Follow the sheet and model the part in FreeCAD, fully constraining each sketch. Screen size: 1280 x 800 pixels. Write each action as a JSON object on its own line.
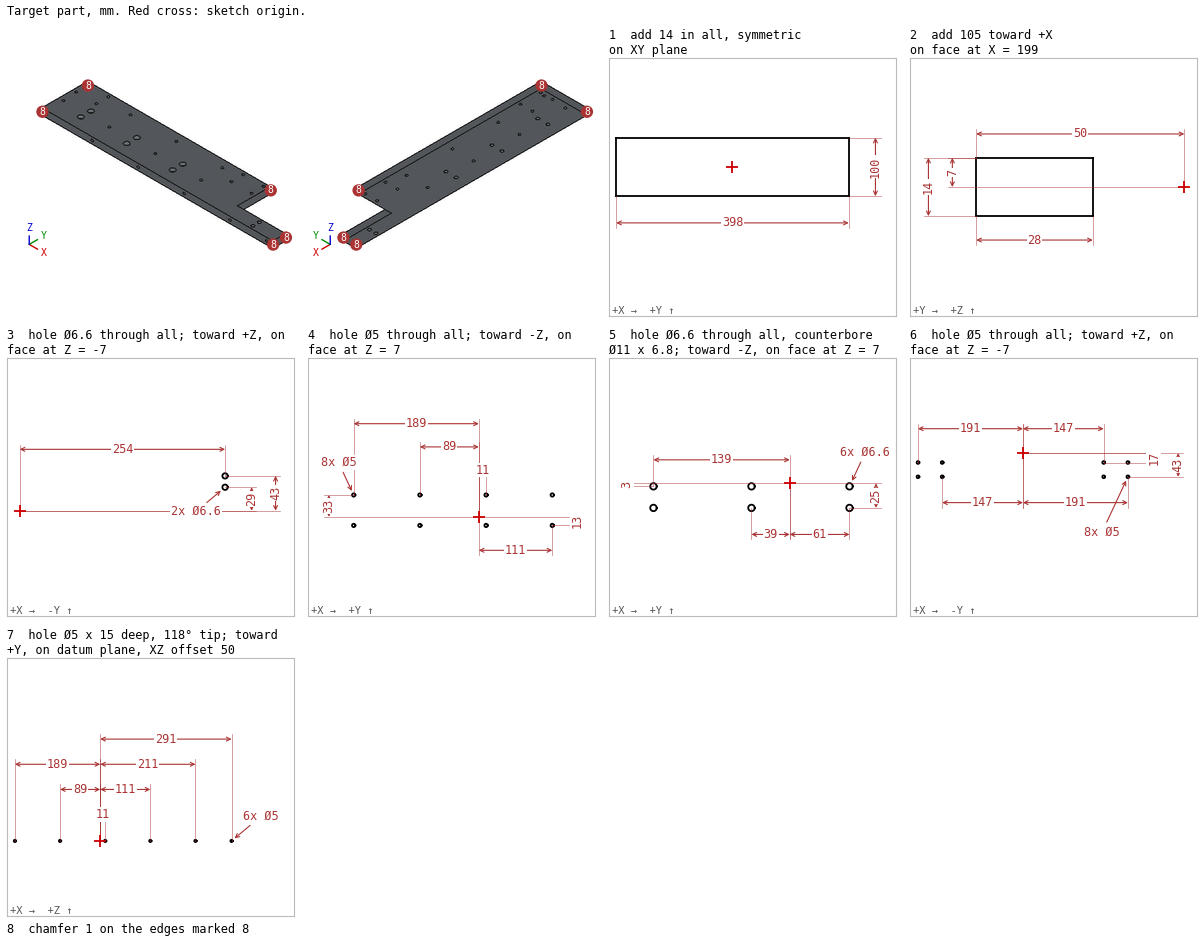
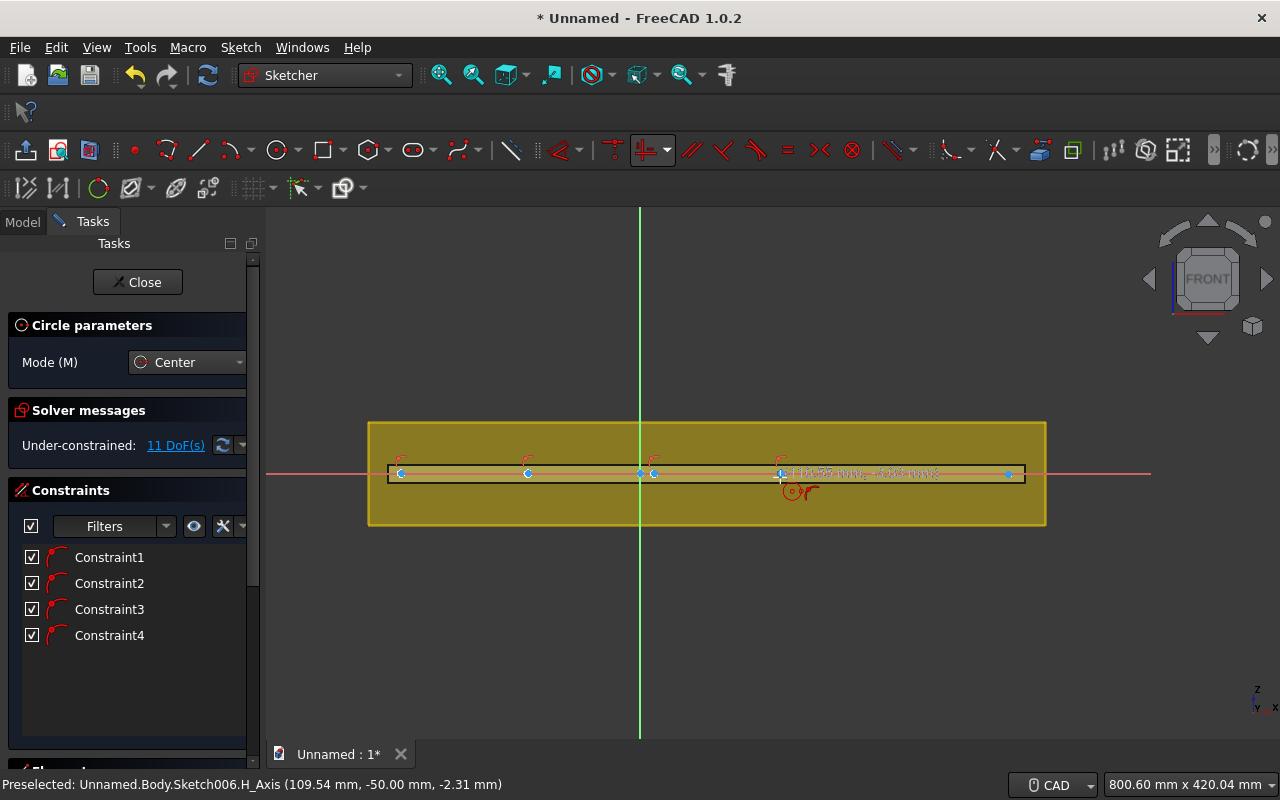
{"action": "scroll", "coordinate": [908, 474], "scroll_direction": "up", "scroll_amount": 10}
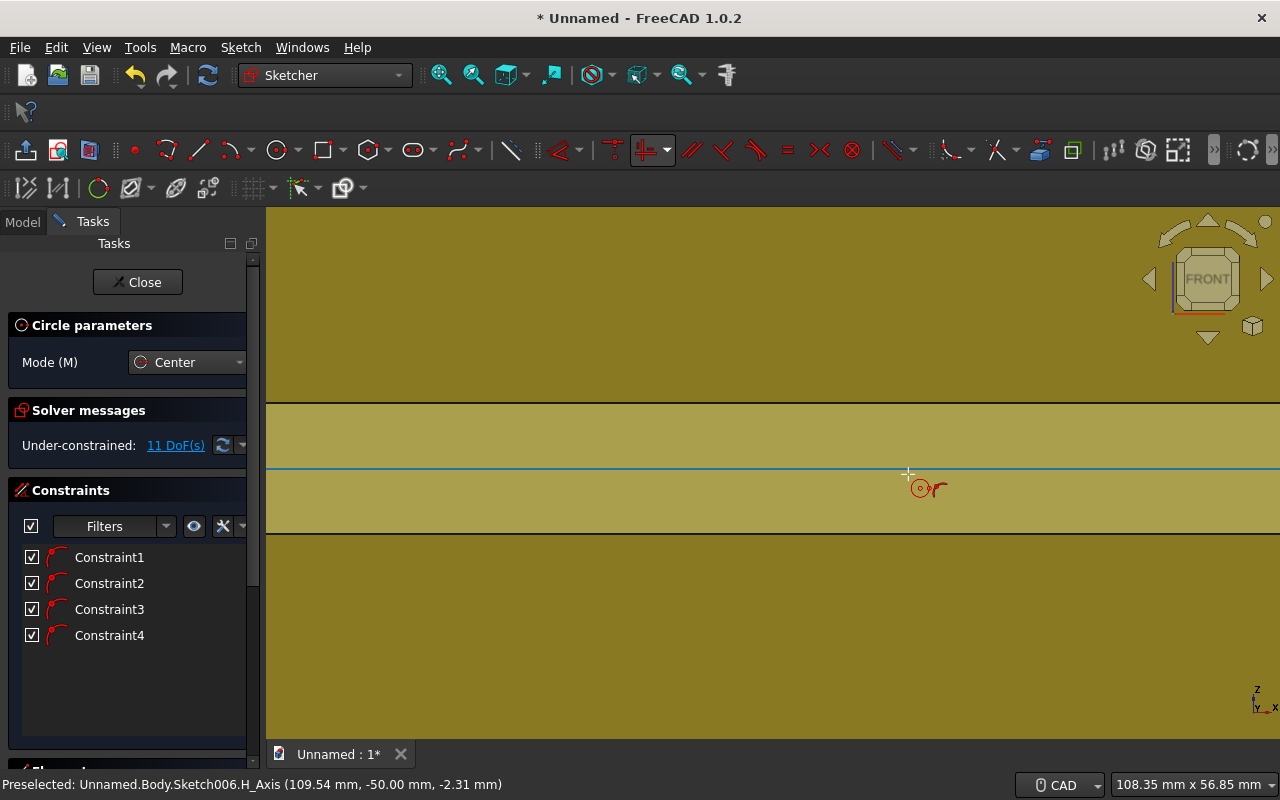
{"action": "scroll", "coordinate": [908, 474], "scroll_direction": "down", "scroll_amount": 10}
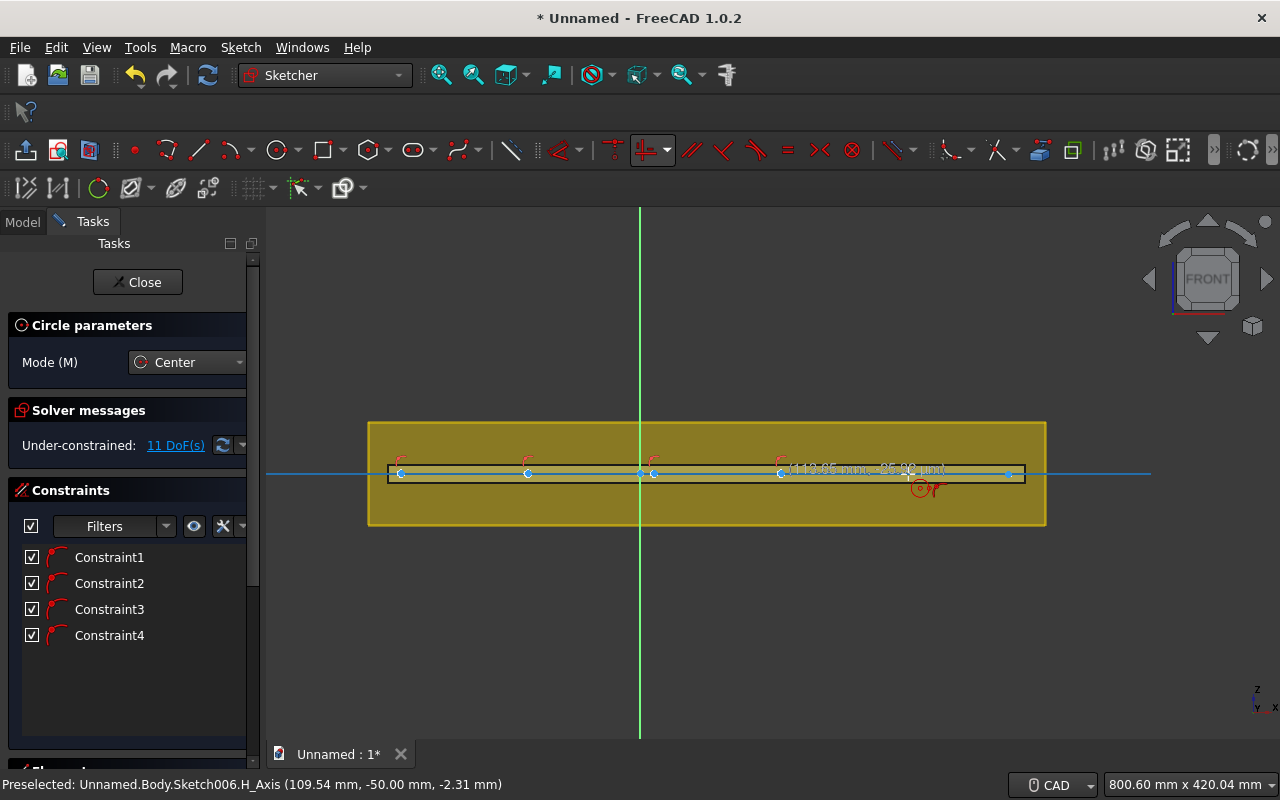
{"action": "left_click", "coordinate": [908, 474]}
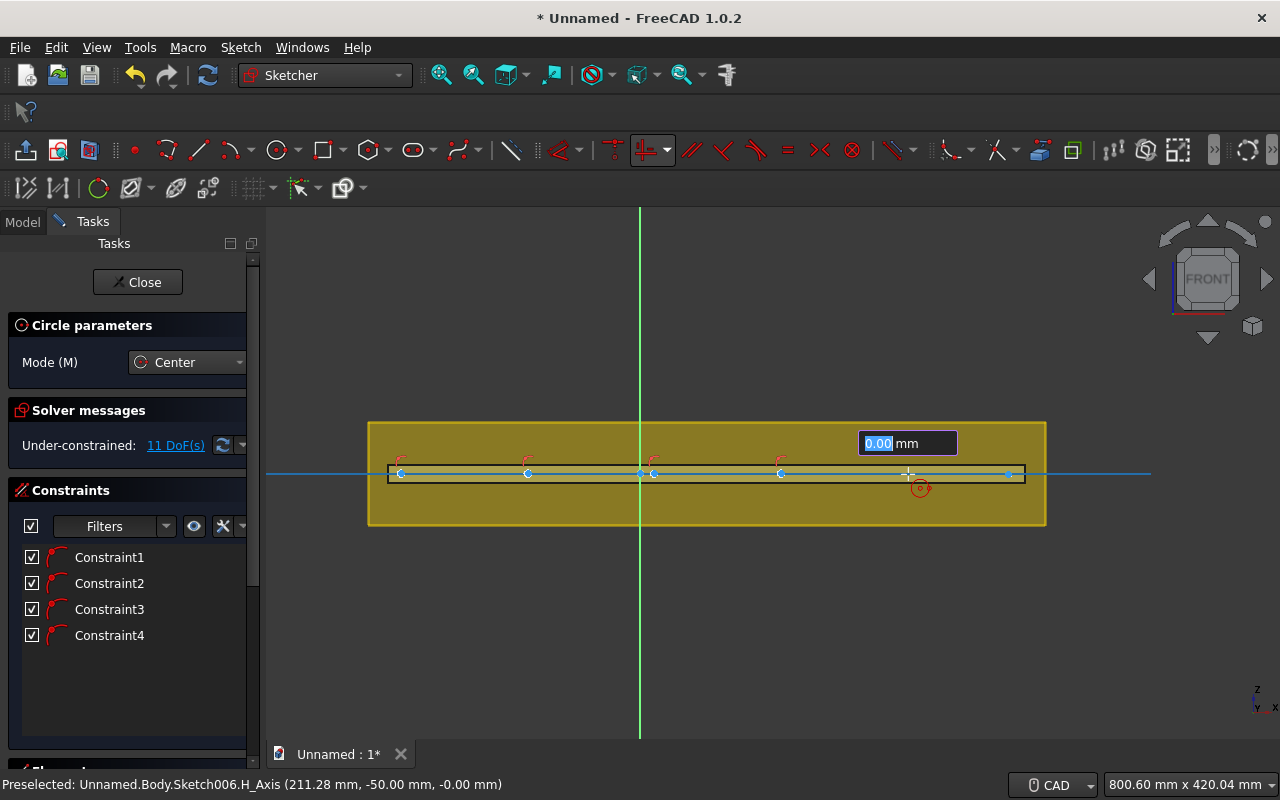
{"action": "scroll", "coordinate": [907, 477], "scroll_direction": "up", "scroll_amount": 9}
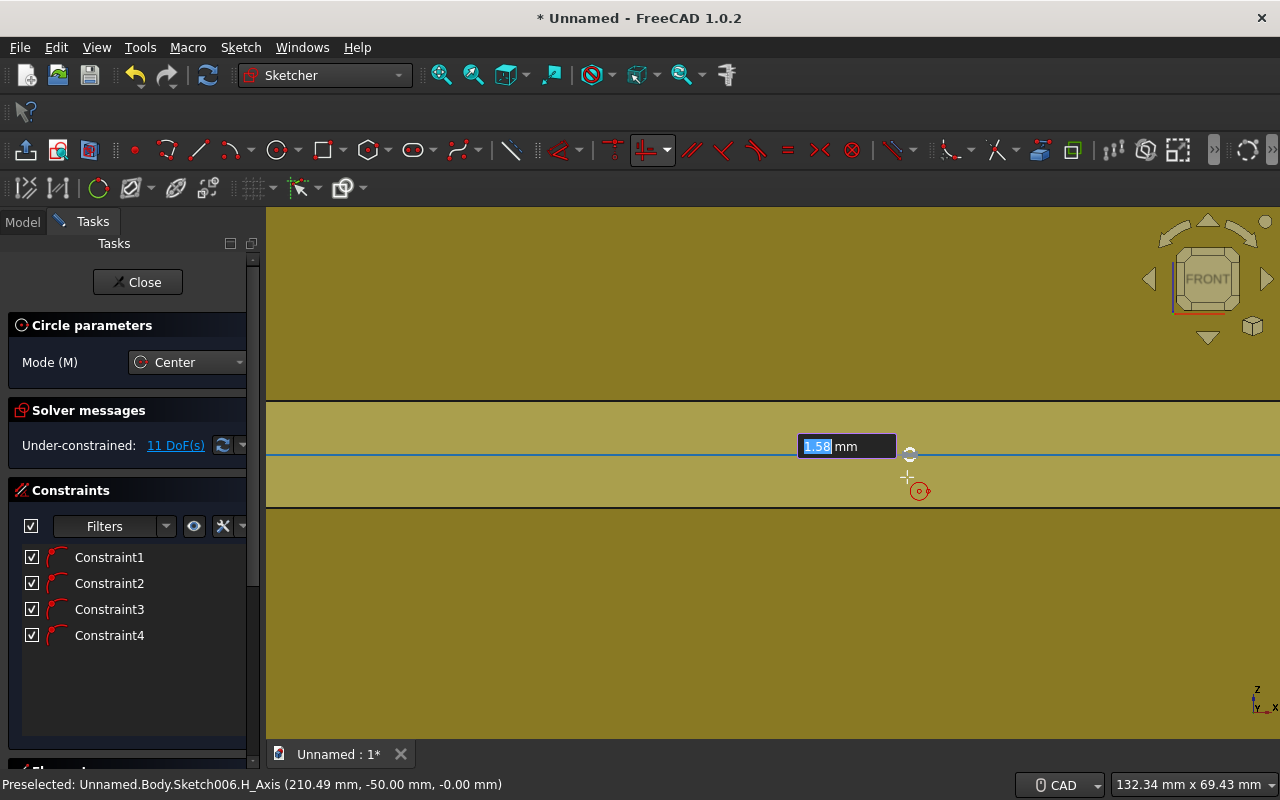
{"action": "left_click", "coordinate": [901, 473]}
{"action": "key", "text": "Escape"}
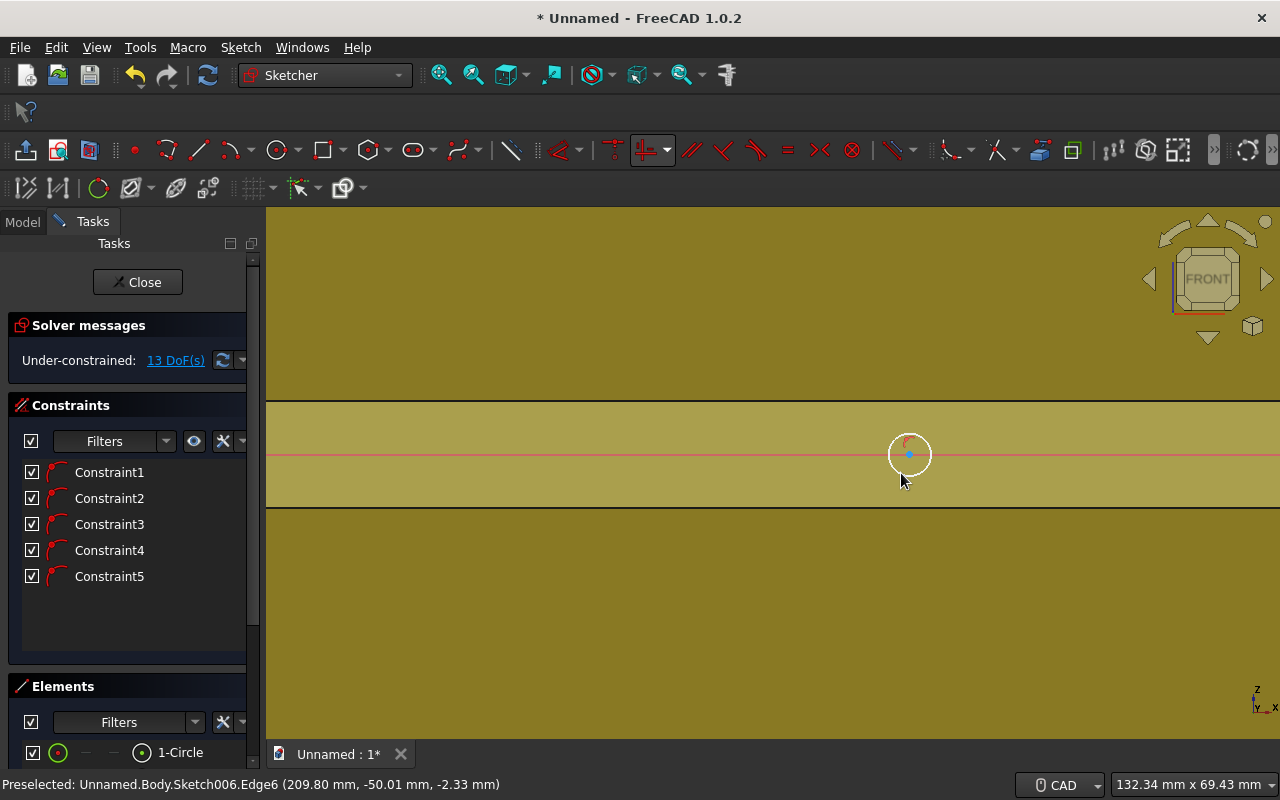
{"action": "scroll", "coordinate": [907, 477], "scroll_direction": "down", "scroll_amount": 9}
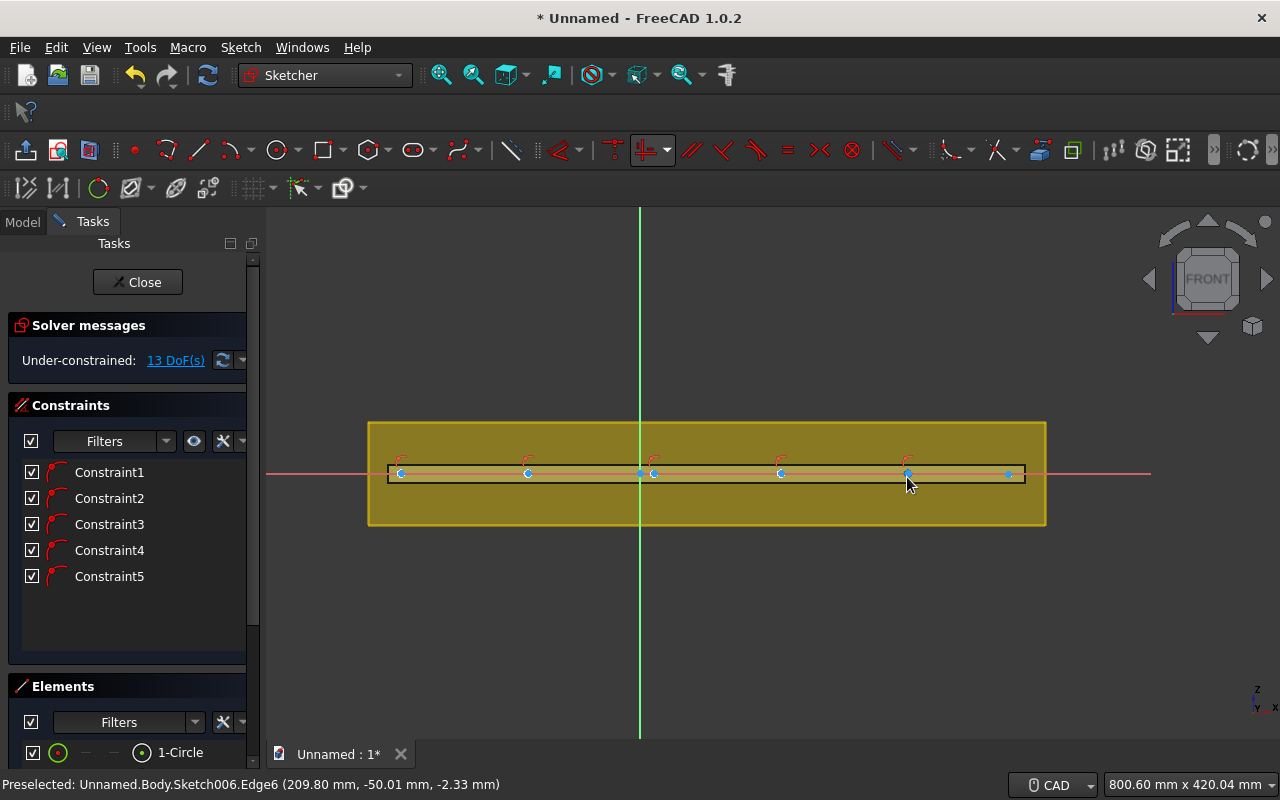
{"action": "scroll", "coordinate": [1011, 473], "scroll_direction": "up", "scroll_amount": 10}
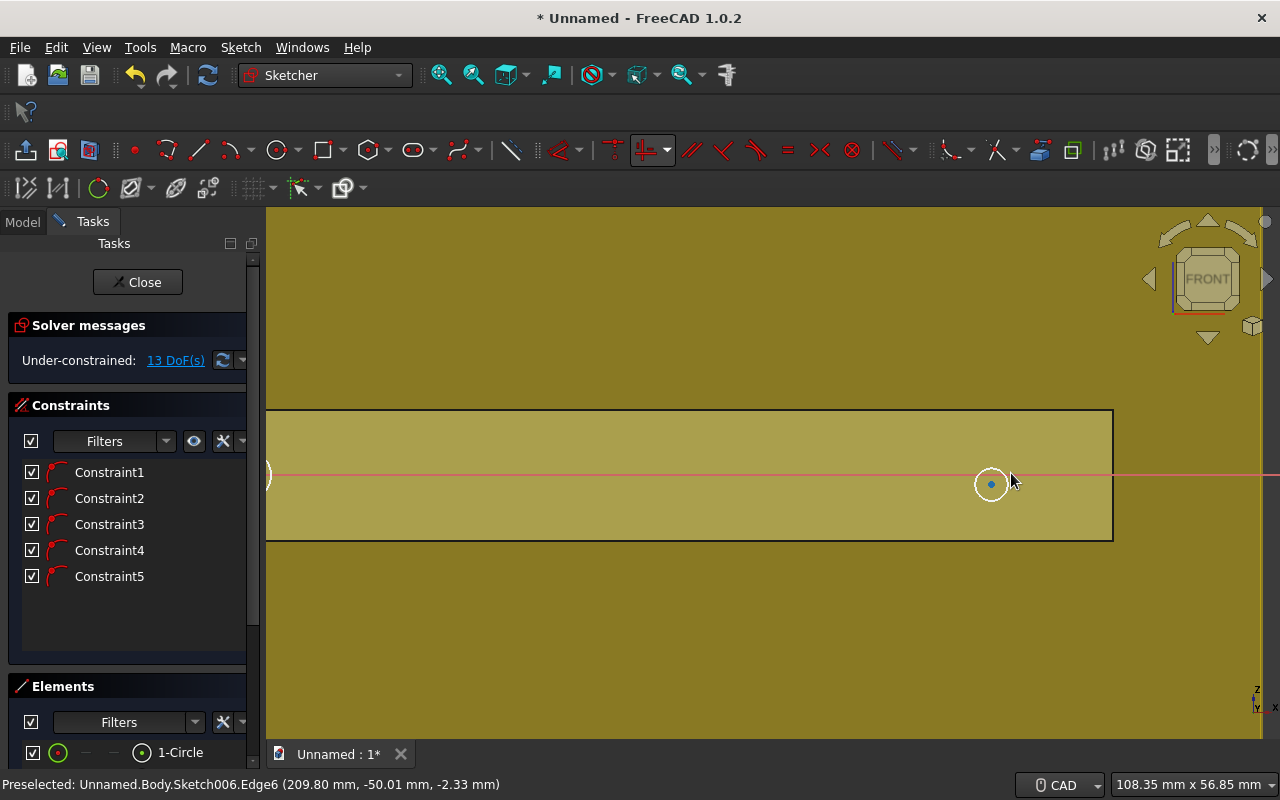
{"action": "left_click", "coordinate": [1003, 473]}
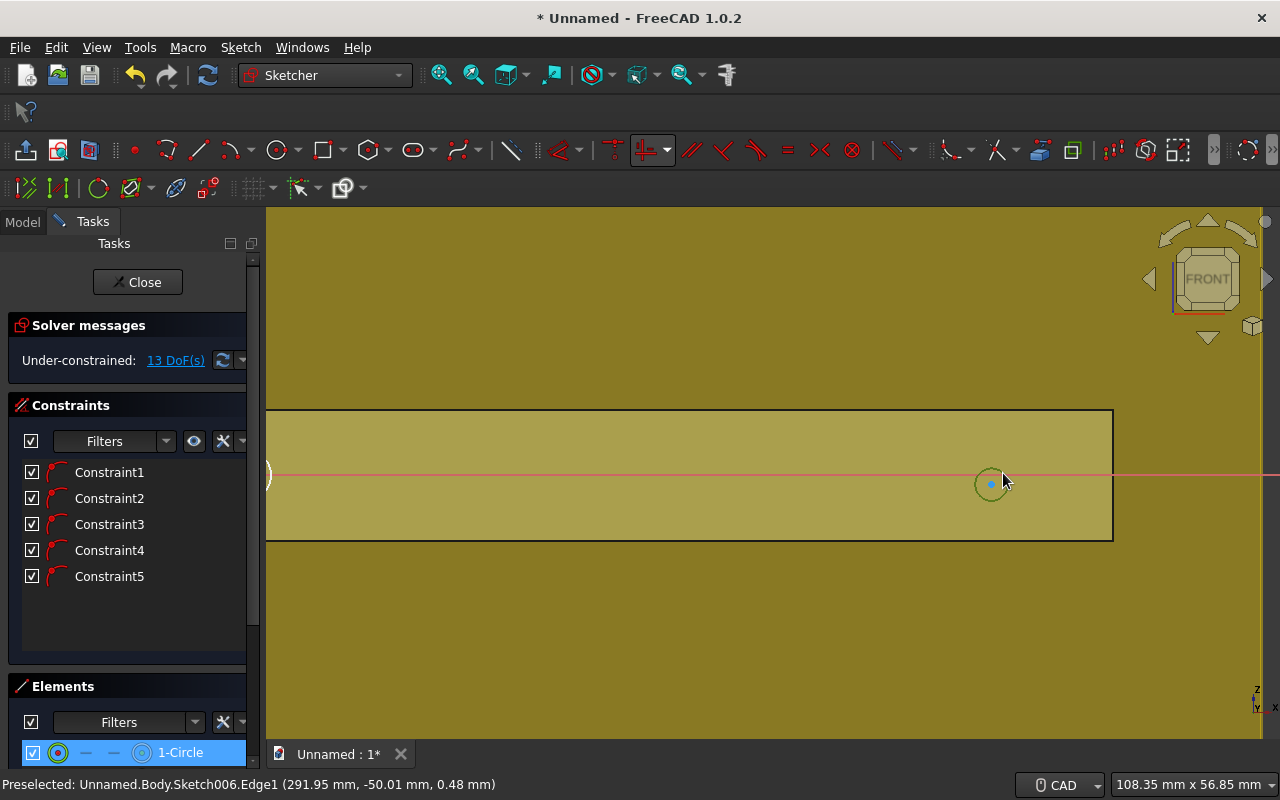
{"action": "scroll", "coordinate": [1011, 473], "scroll_direction": "down", "scroll_amount": 10}